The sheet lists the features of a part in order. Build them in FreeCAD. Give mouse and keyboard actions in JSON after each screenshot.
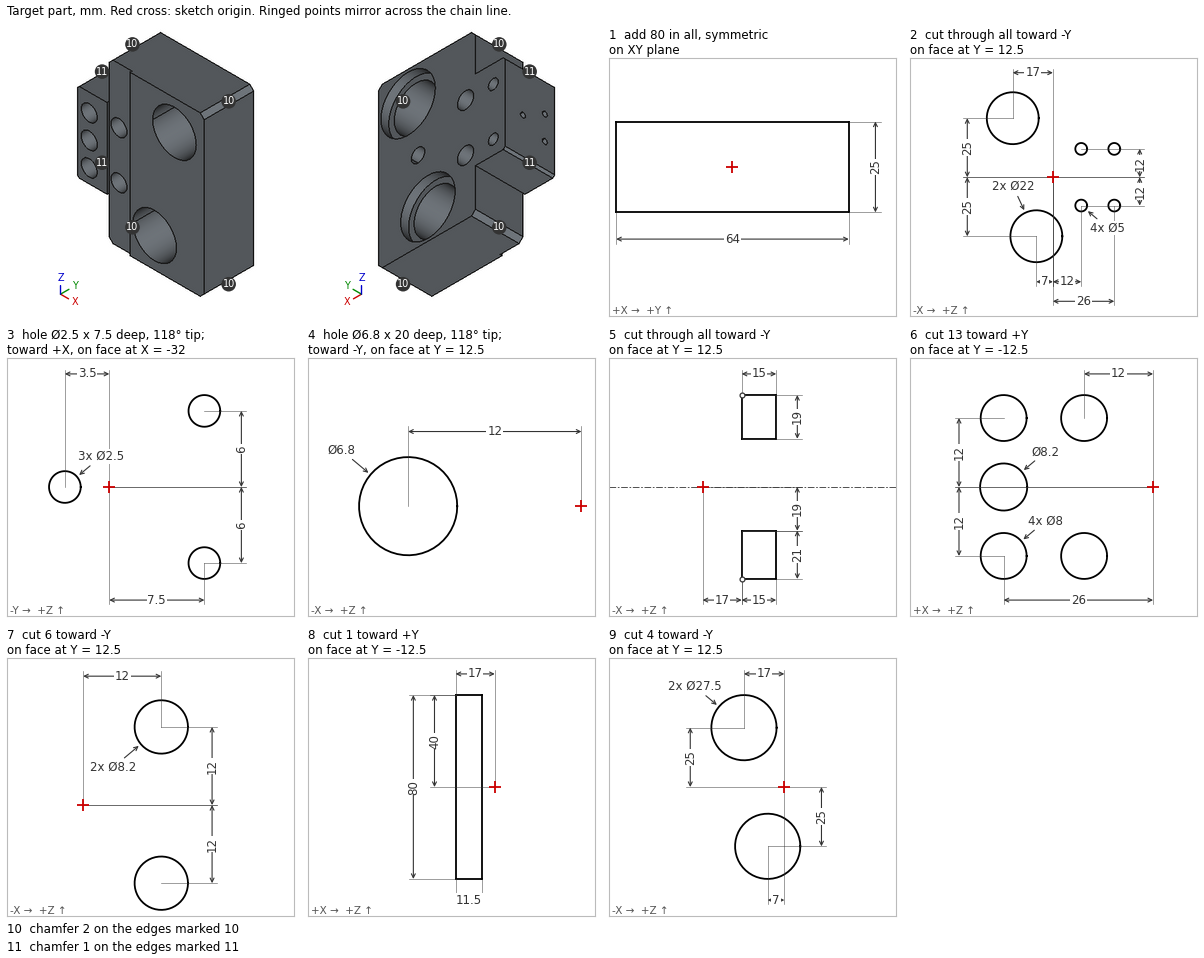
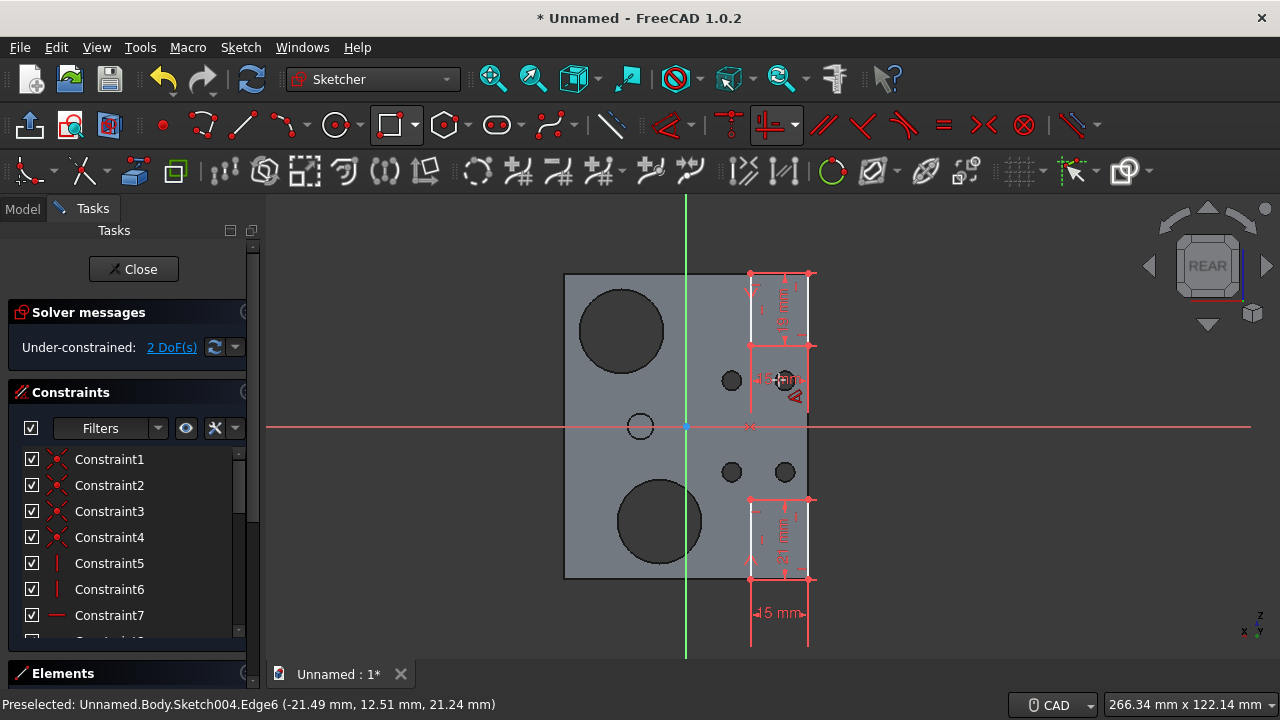
{"action": "left_click", "coordinate": [751, 500]}
{"action": "left_click", "coordinate": [704, 534]}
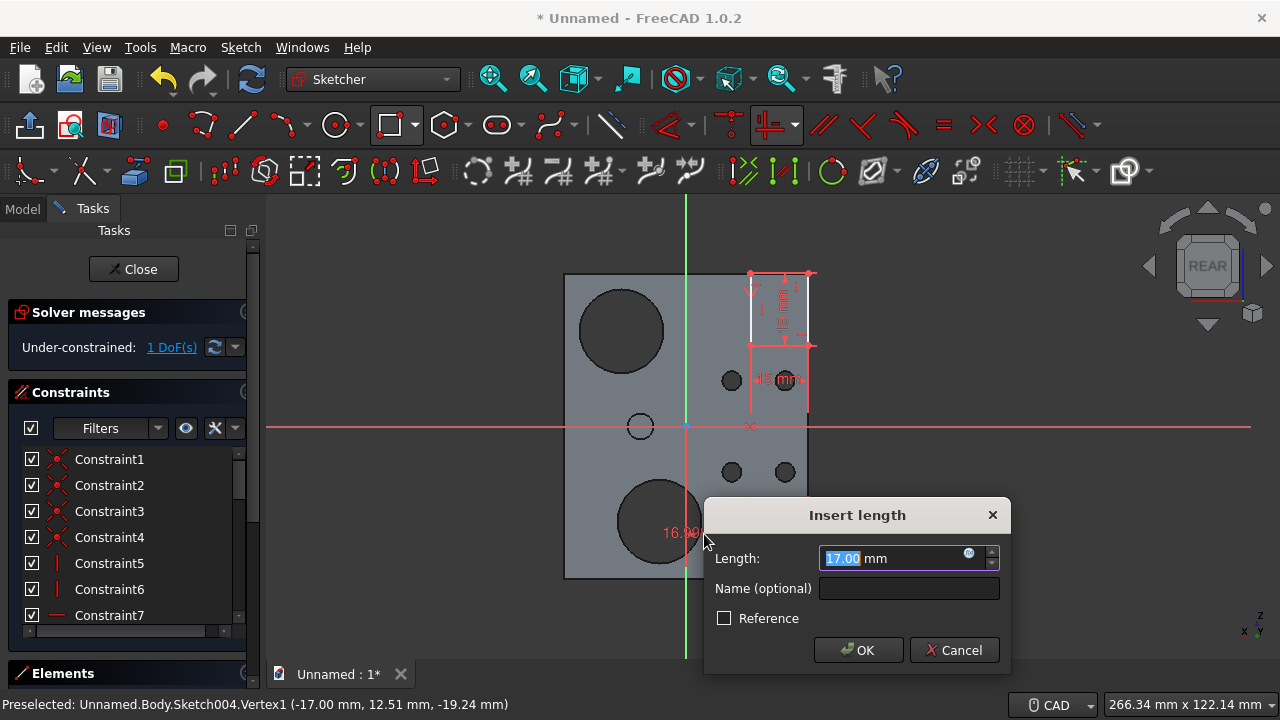
{"action": "type", "text": "17"}
{"action": "key", "text": "Return"}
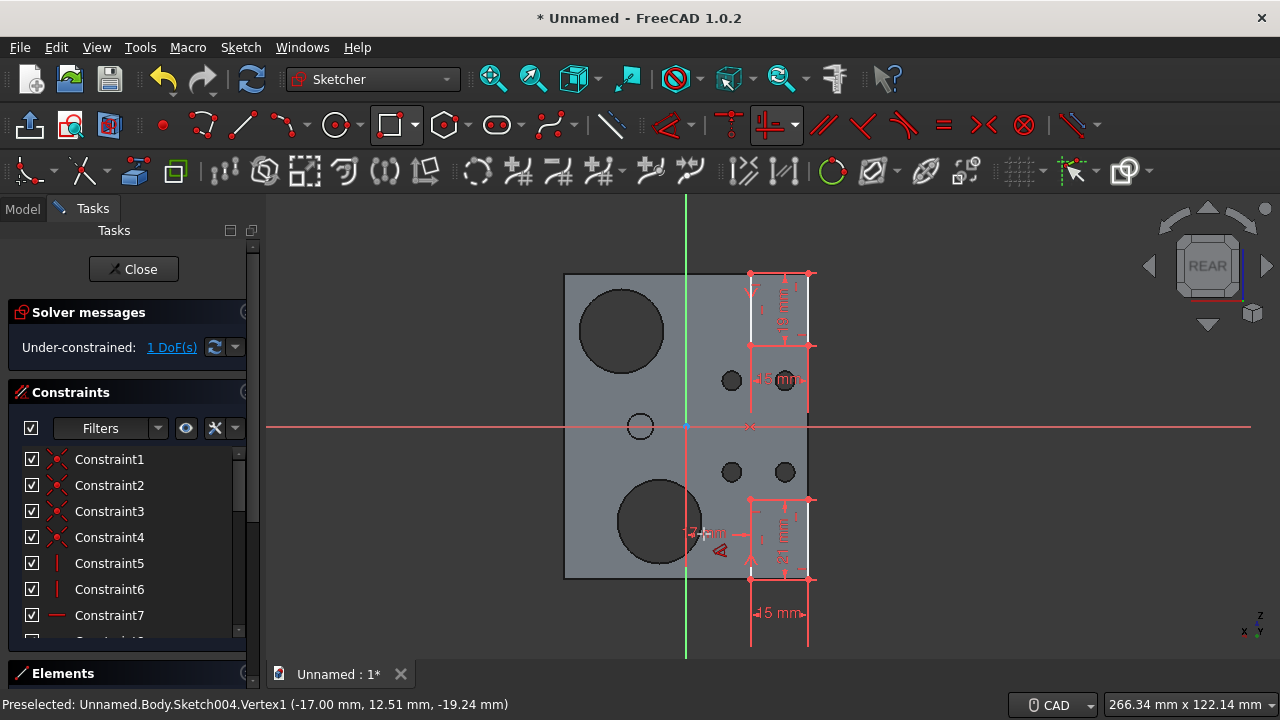
{"action": "left_click", "coordinate": [751, 500]}
{"action": "left_click", "coordinate": [652, 463]}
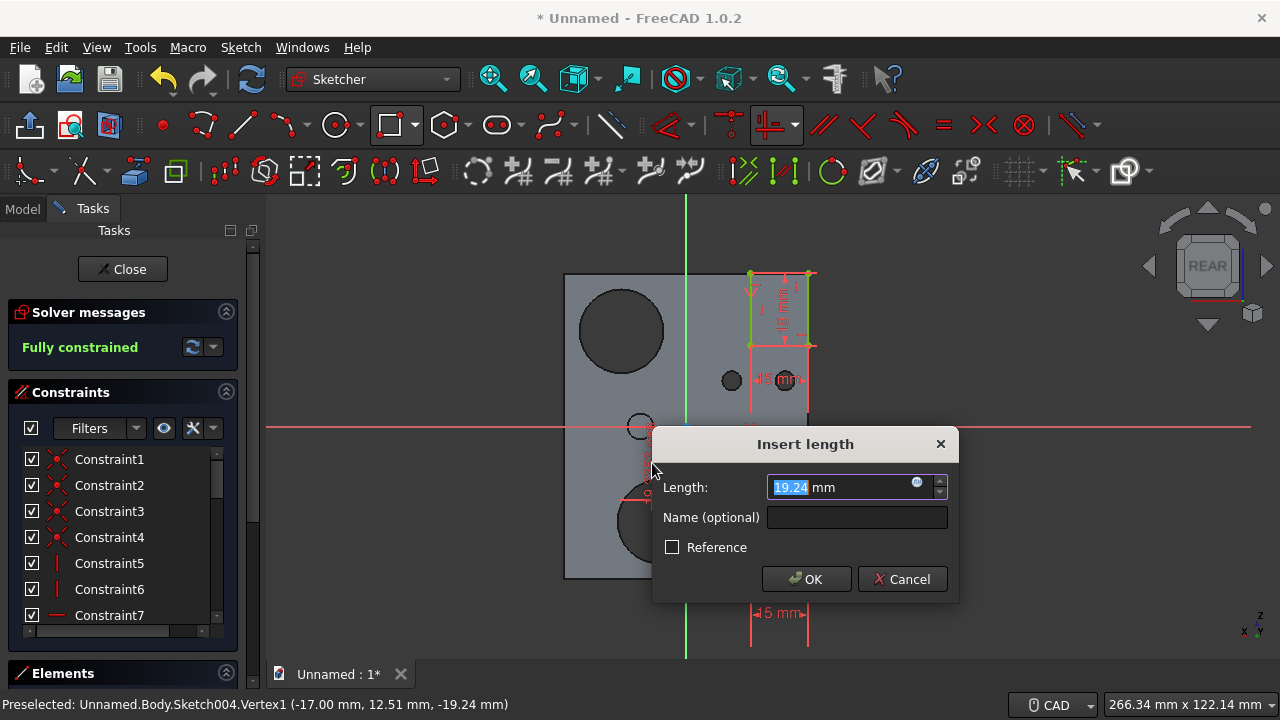
{"action": "type", "text": "19"}
{"action": "key", "text": "Return"}
{"action": "key", "text": "Escape"}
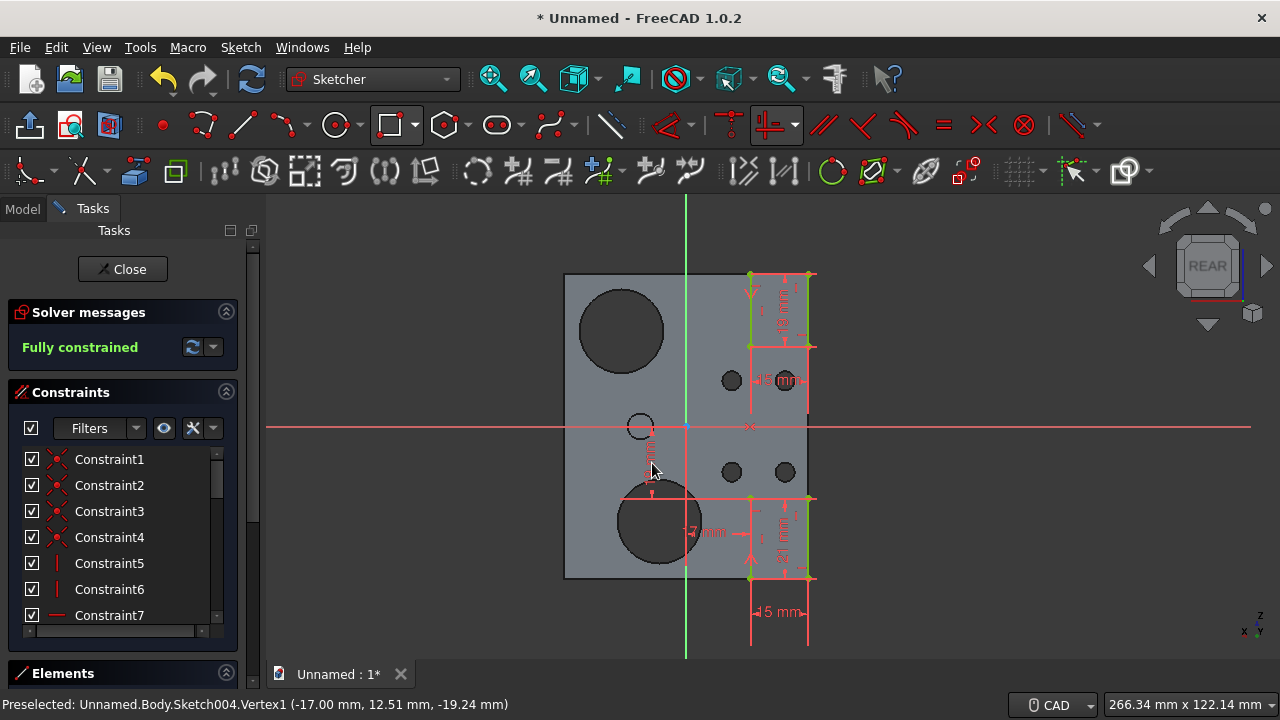
{"action": "left_click", "coordinate": [123, 269]}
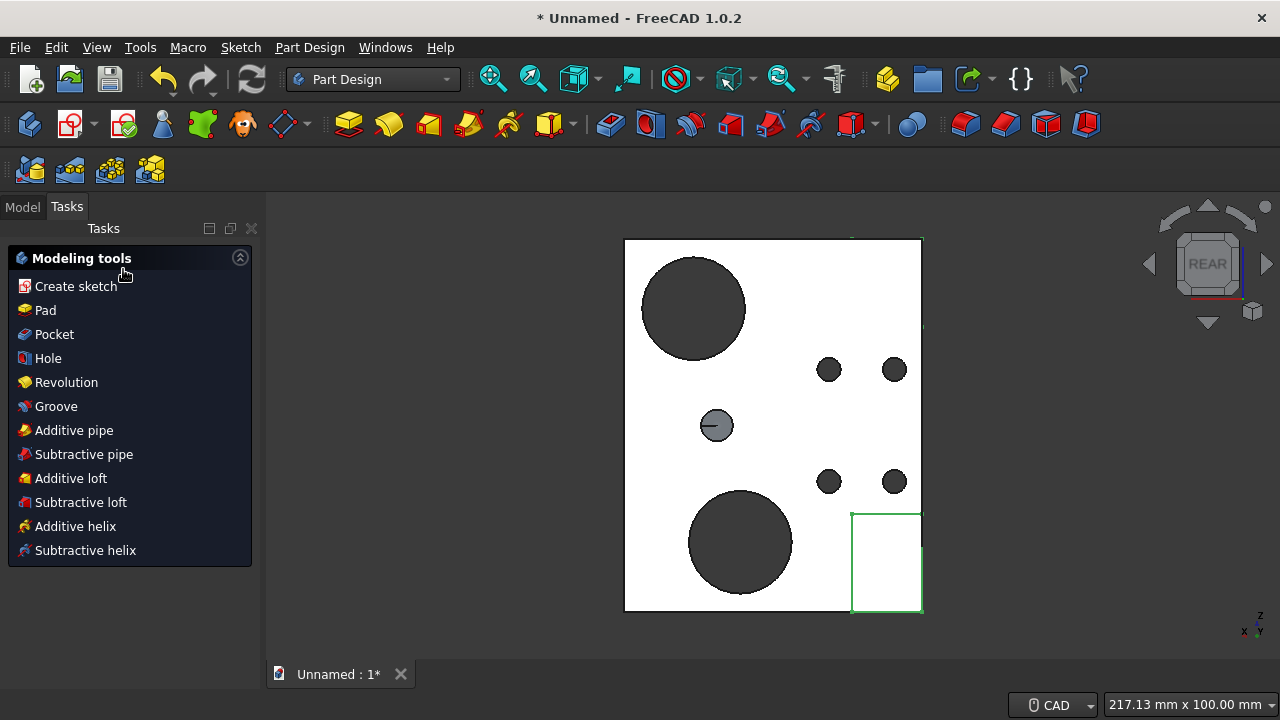
{"action": "left_click", "coordinate": [612, 124]}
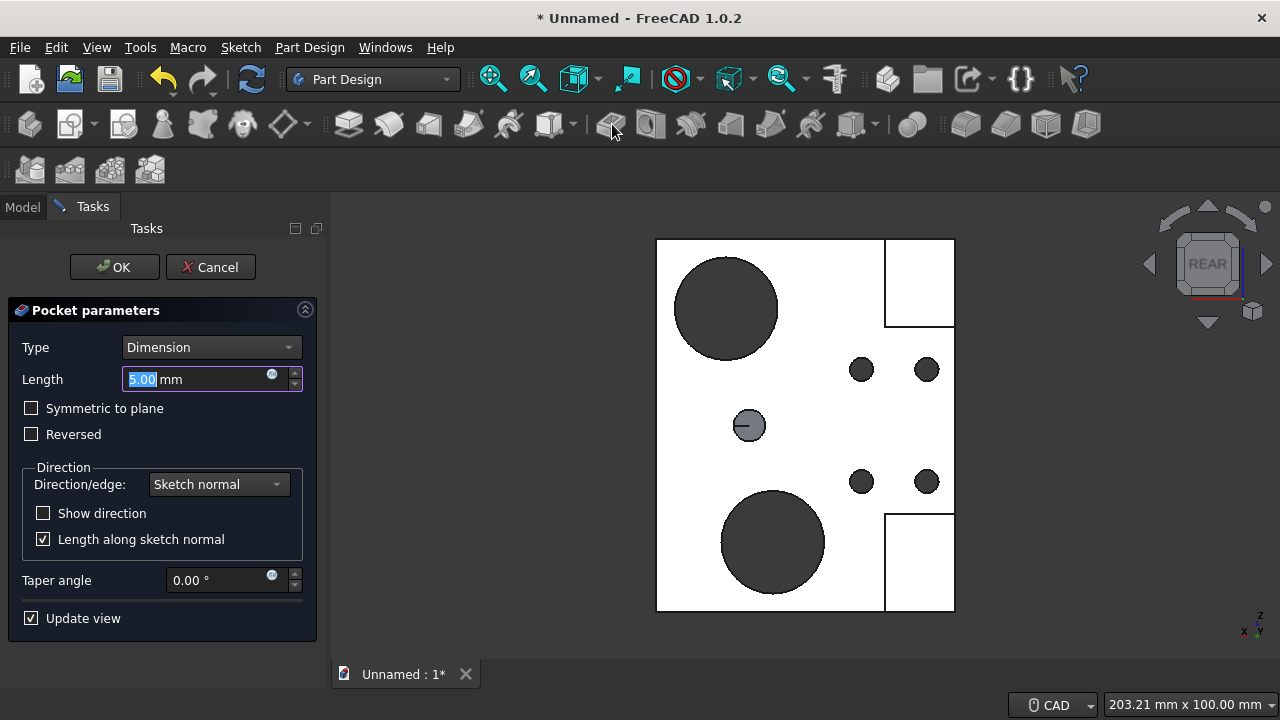
{"action": "left_click", "coordinate": [212, 348]}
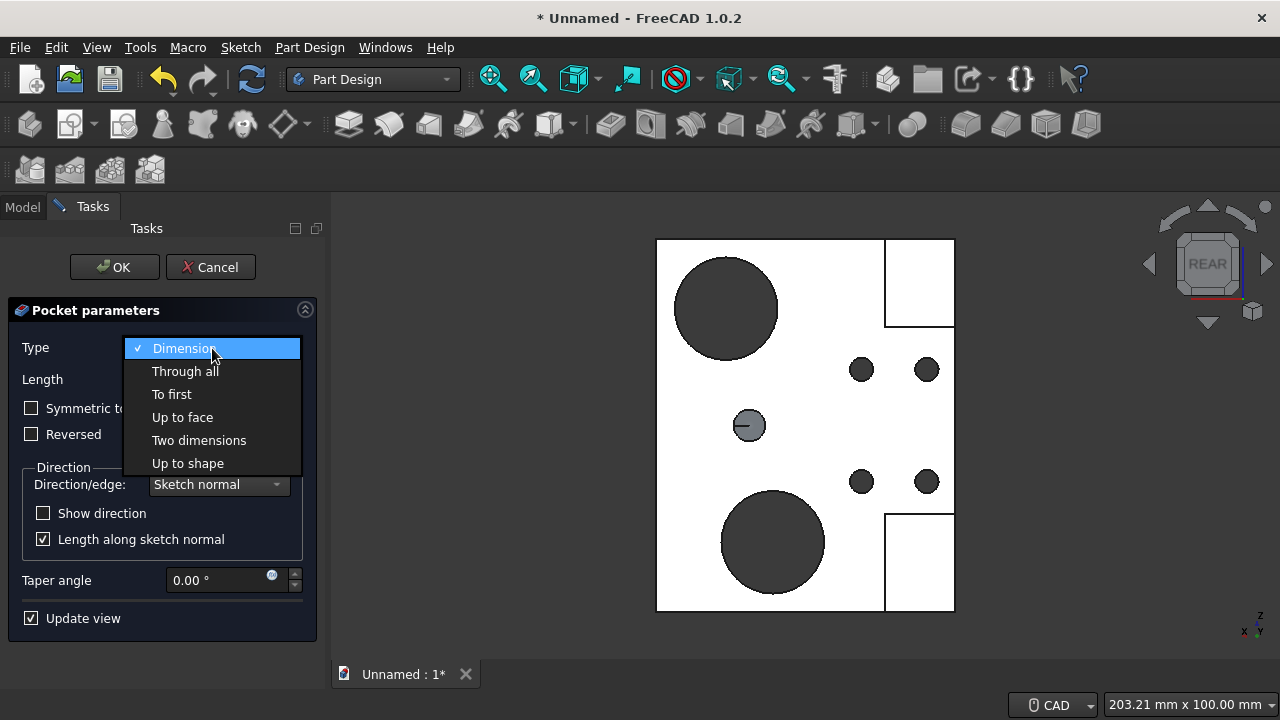
{"action": "left_click", "coordinate": [212, 372]}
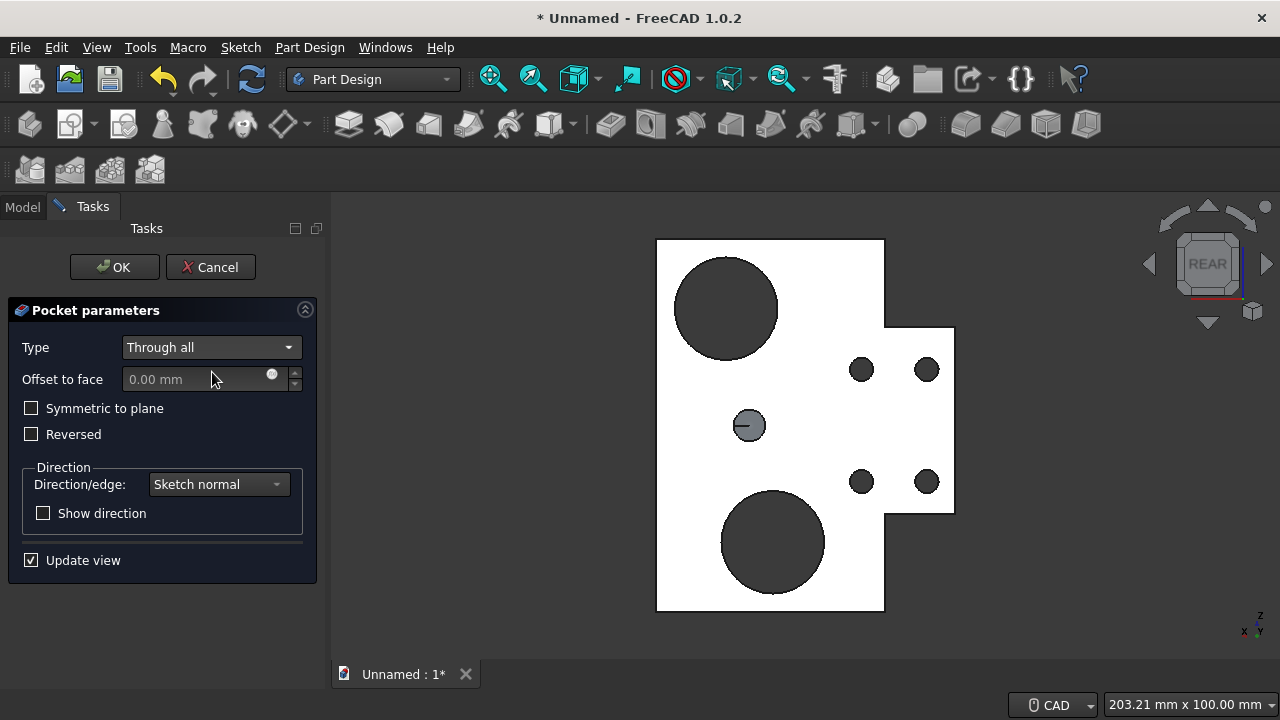
{"action": "left_click", "coordinate": [115, 267]}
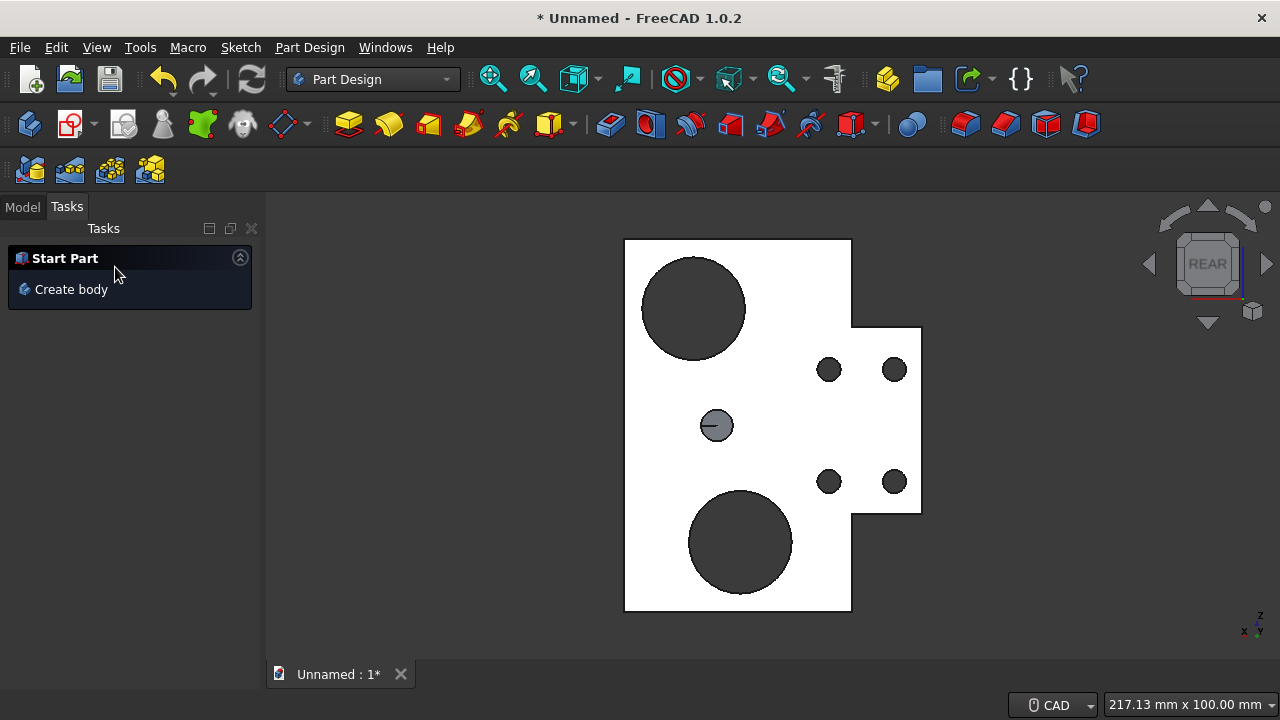
{"action": "key", "text": "0"}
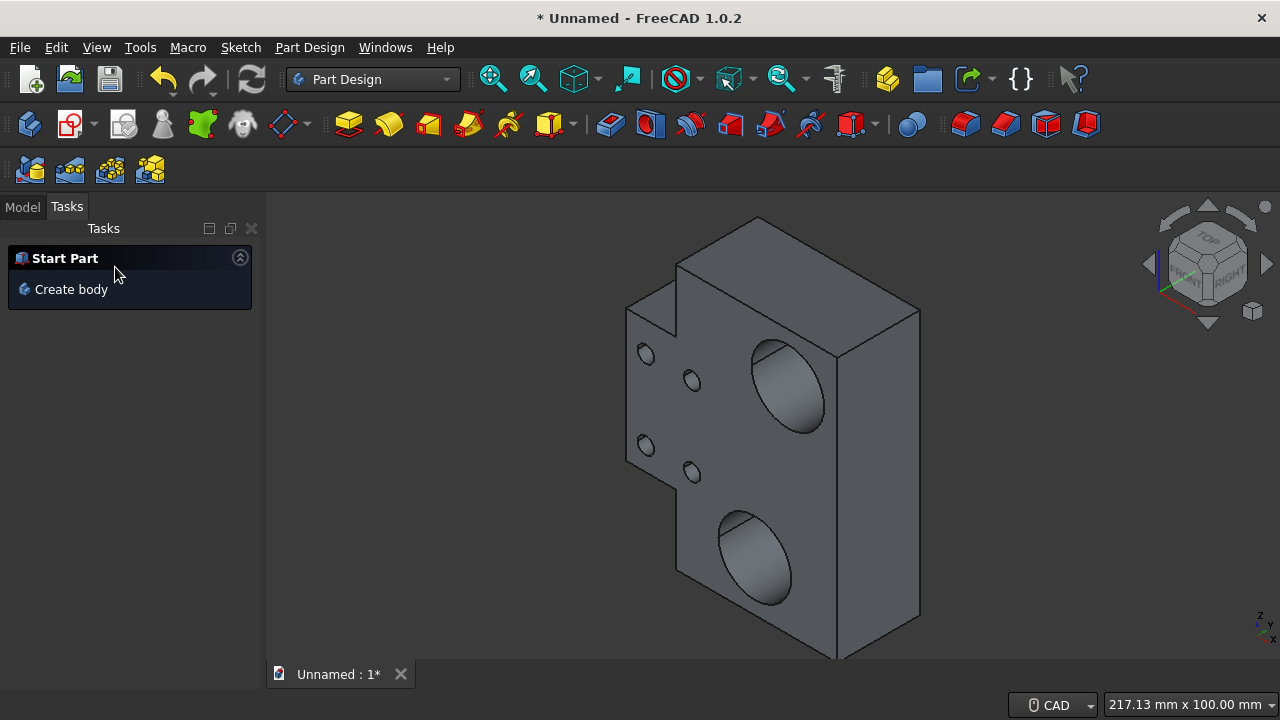
{"action": "left_click", "coordinate": [494, 80]}